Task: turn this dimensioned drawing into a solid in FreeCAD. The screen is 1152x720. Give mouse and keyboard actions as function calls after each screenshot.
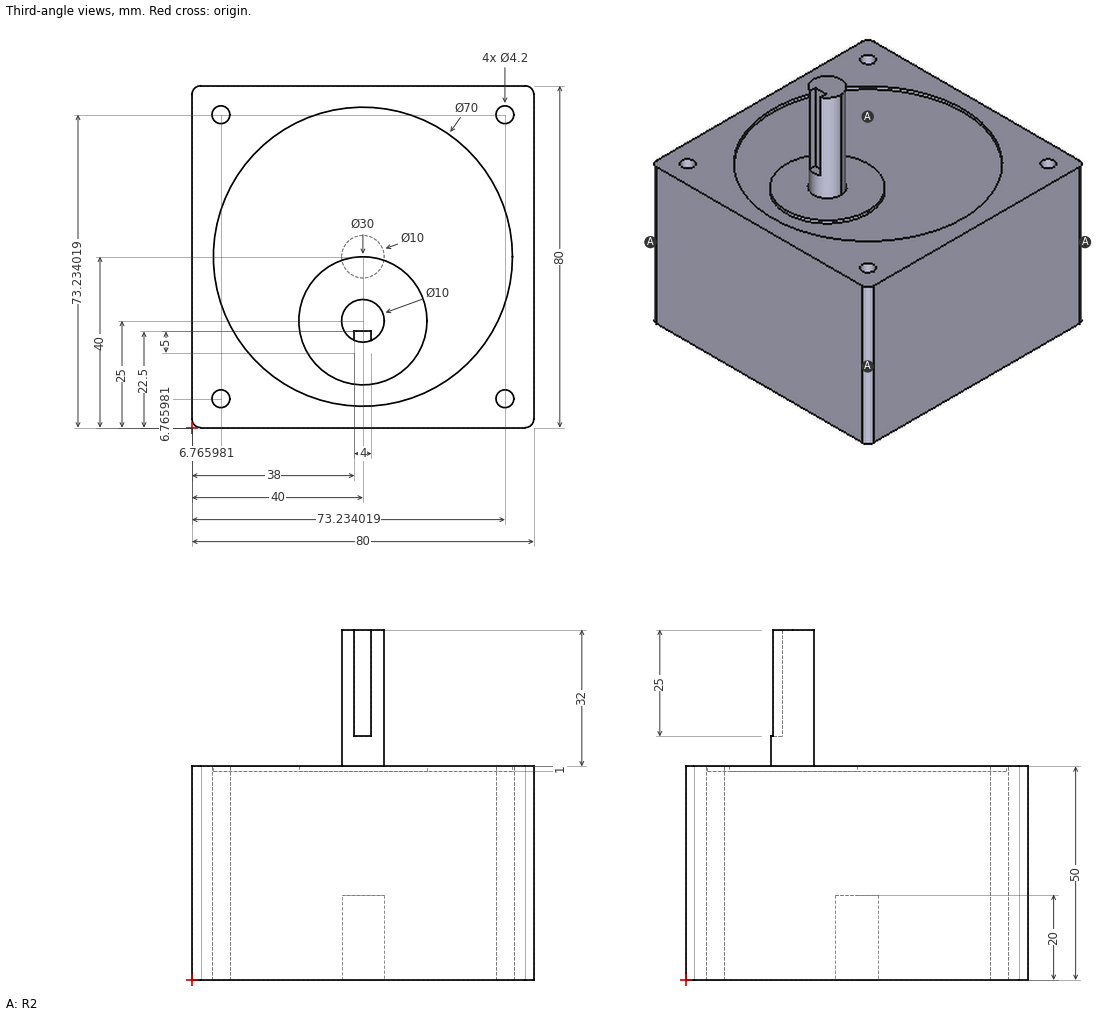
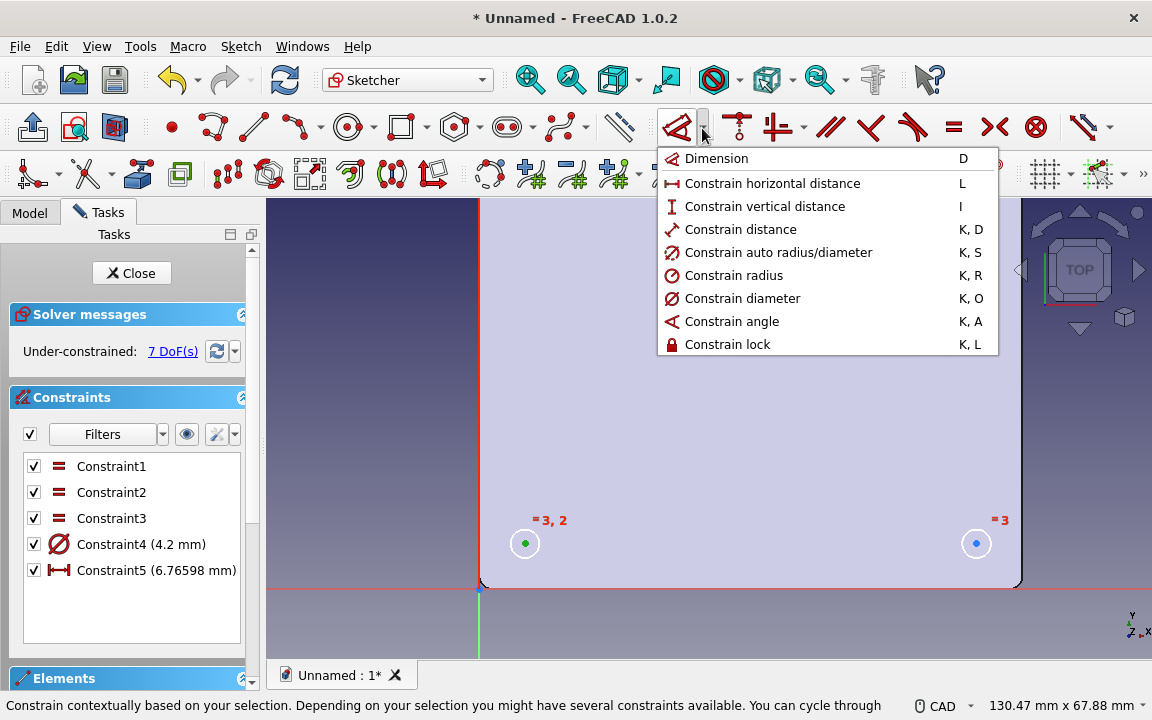
click(828, 184)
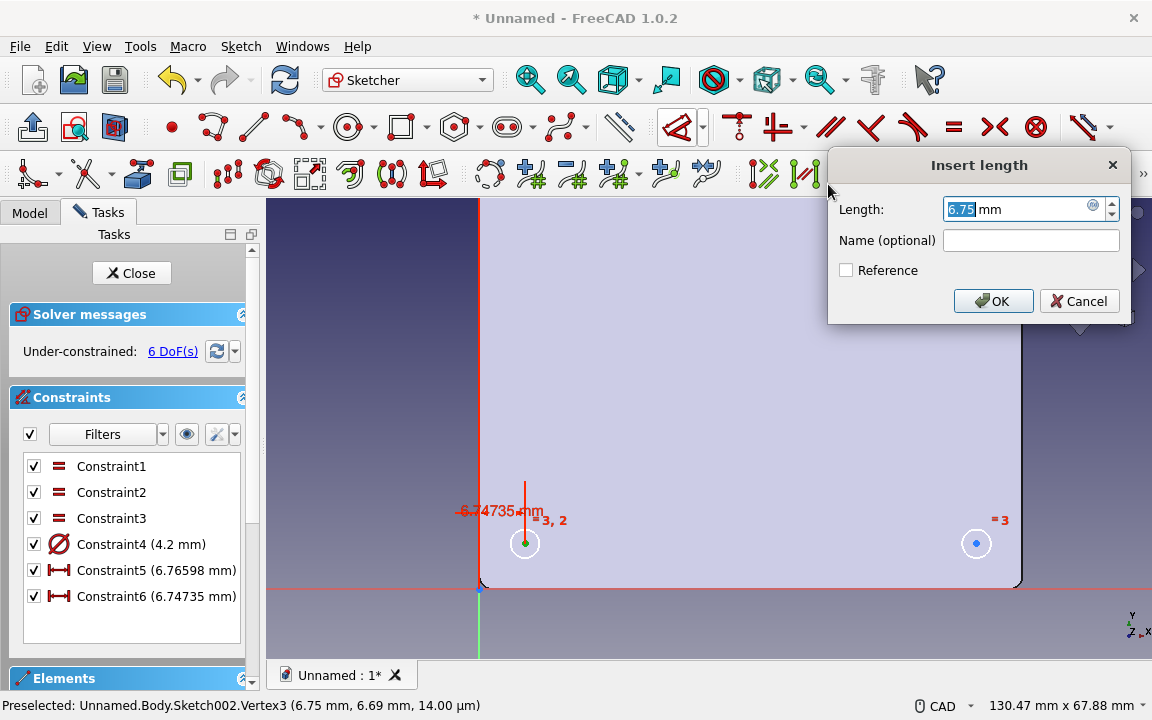
text(6.765981)
key(Return)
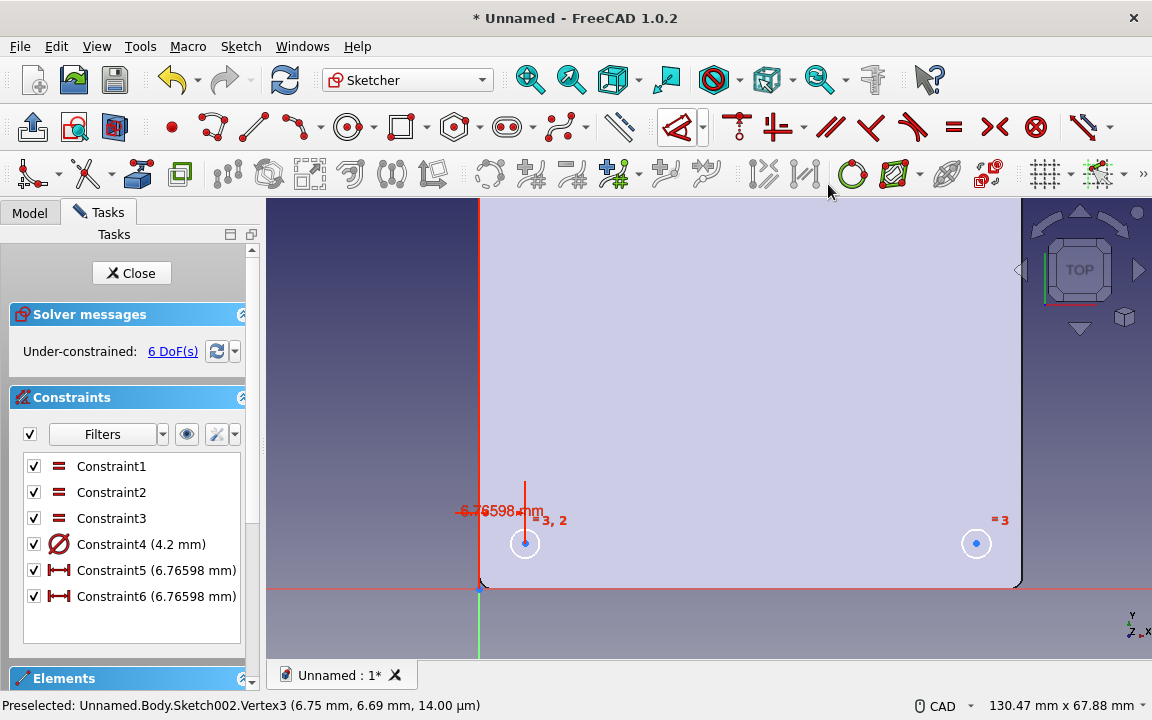
click(525, 544)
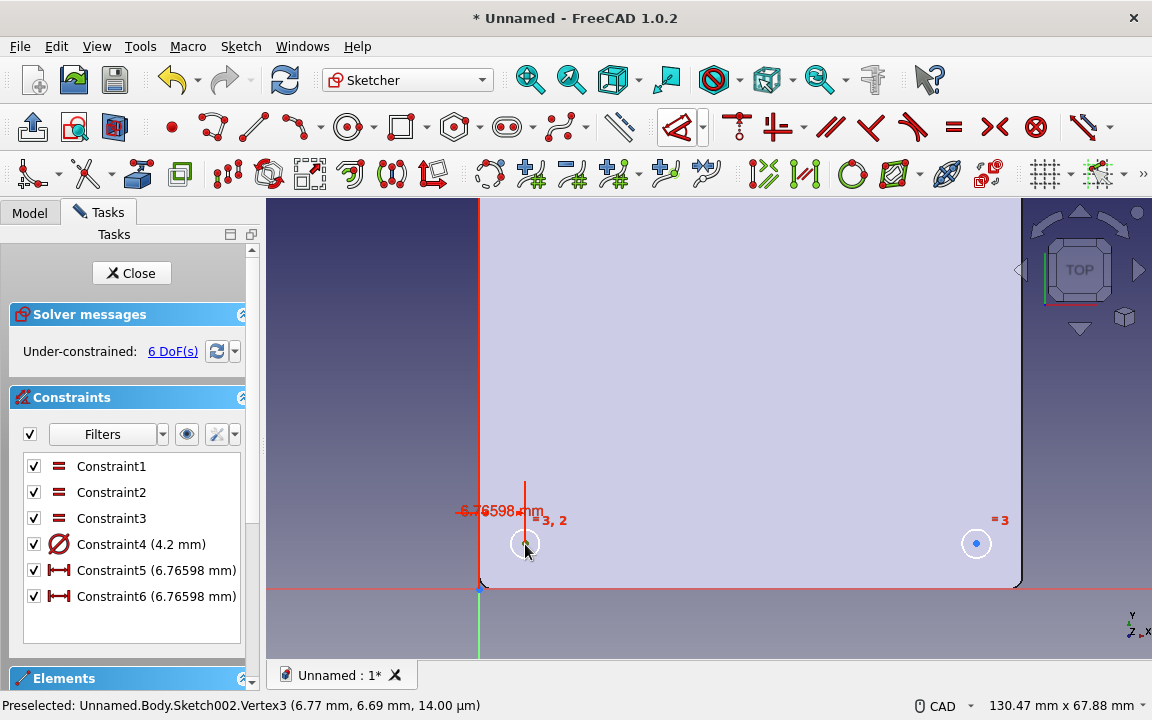
key(i)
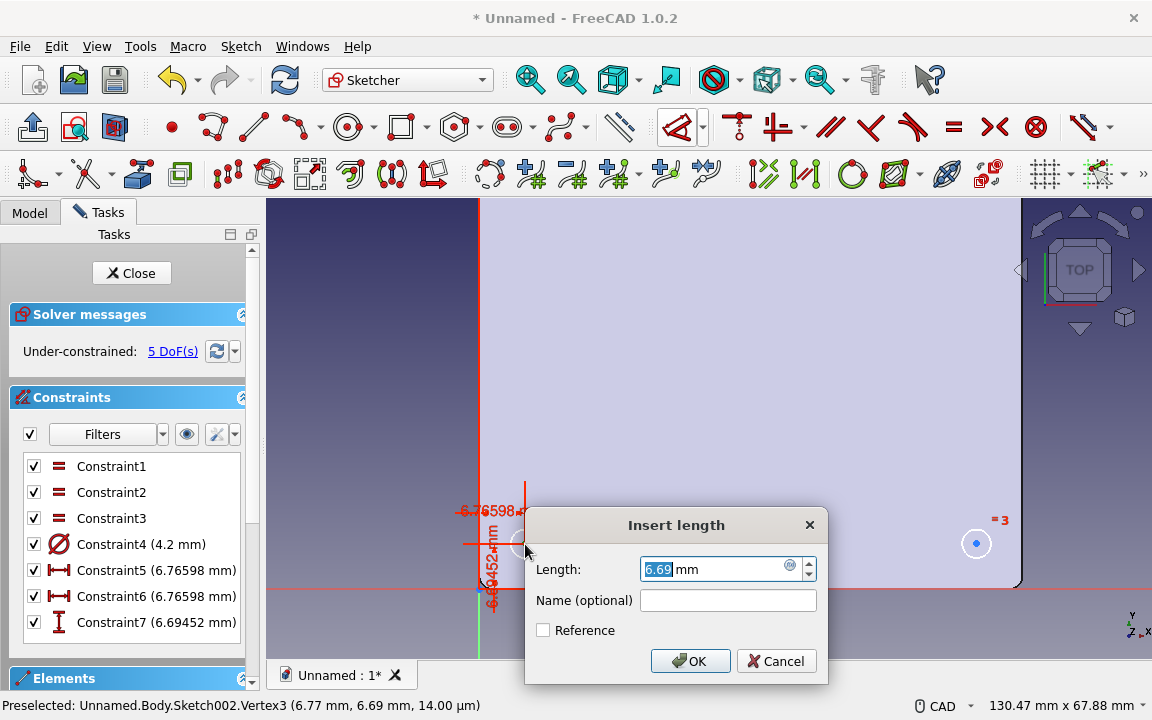
text(6.765981)
key(Return)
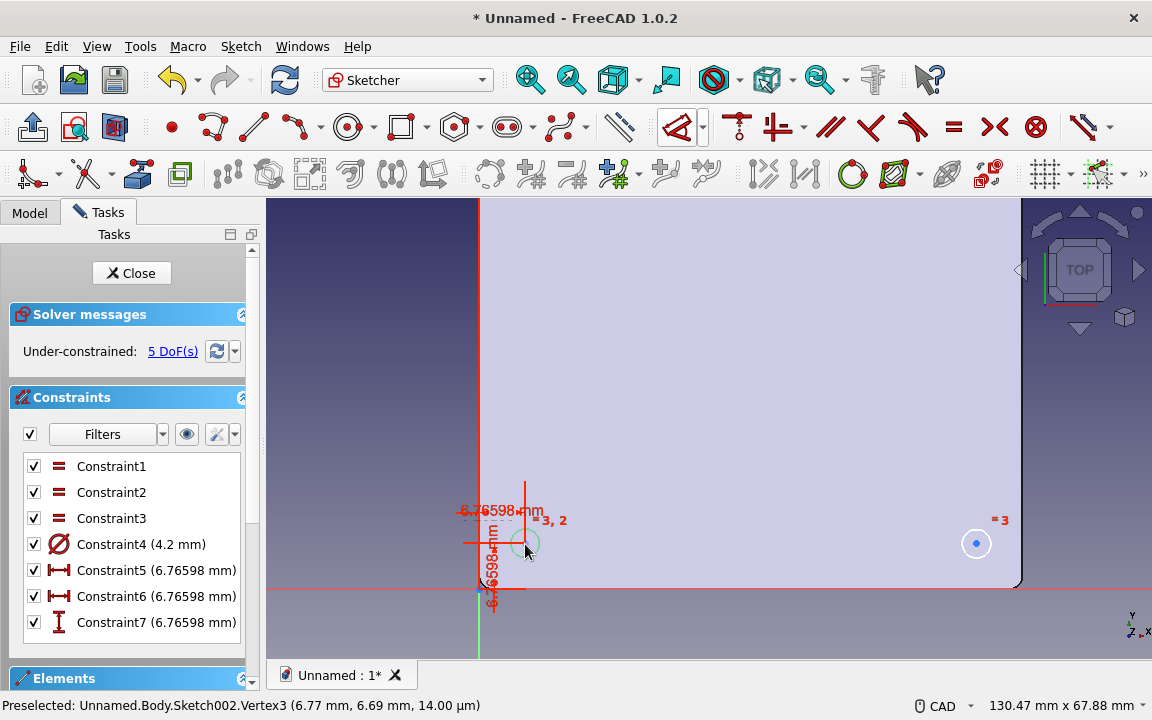
click(977, 544)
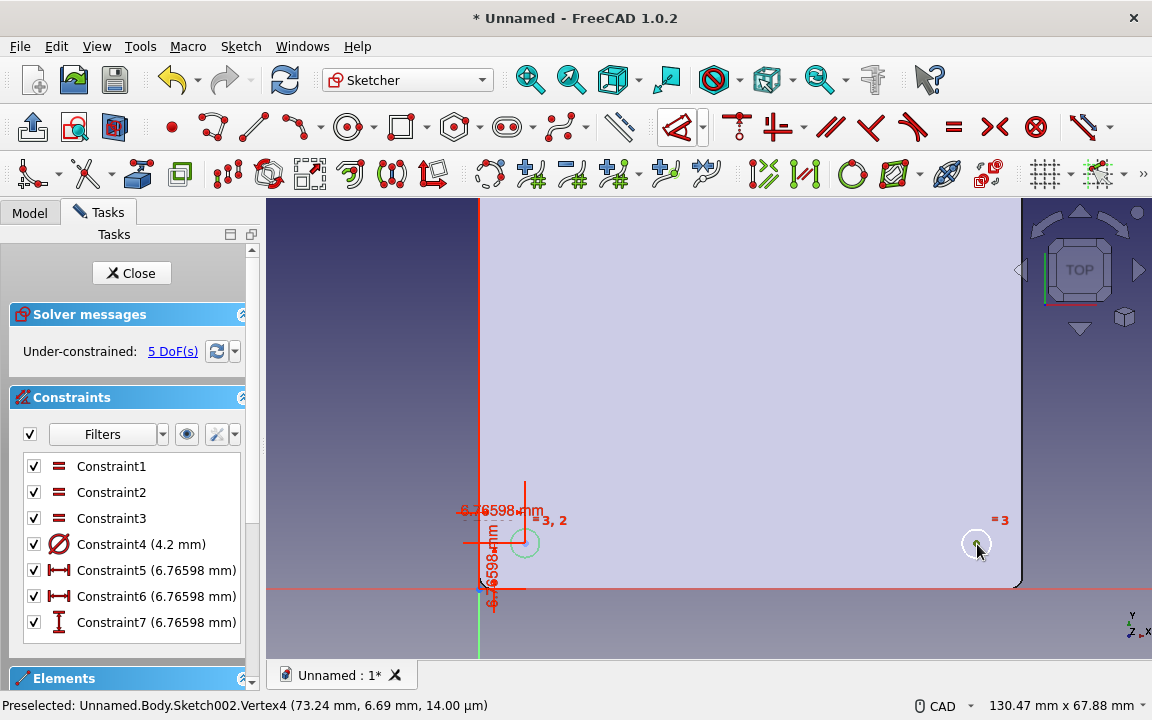
key(i)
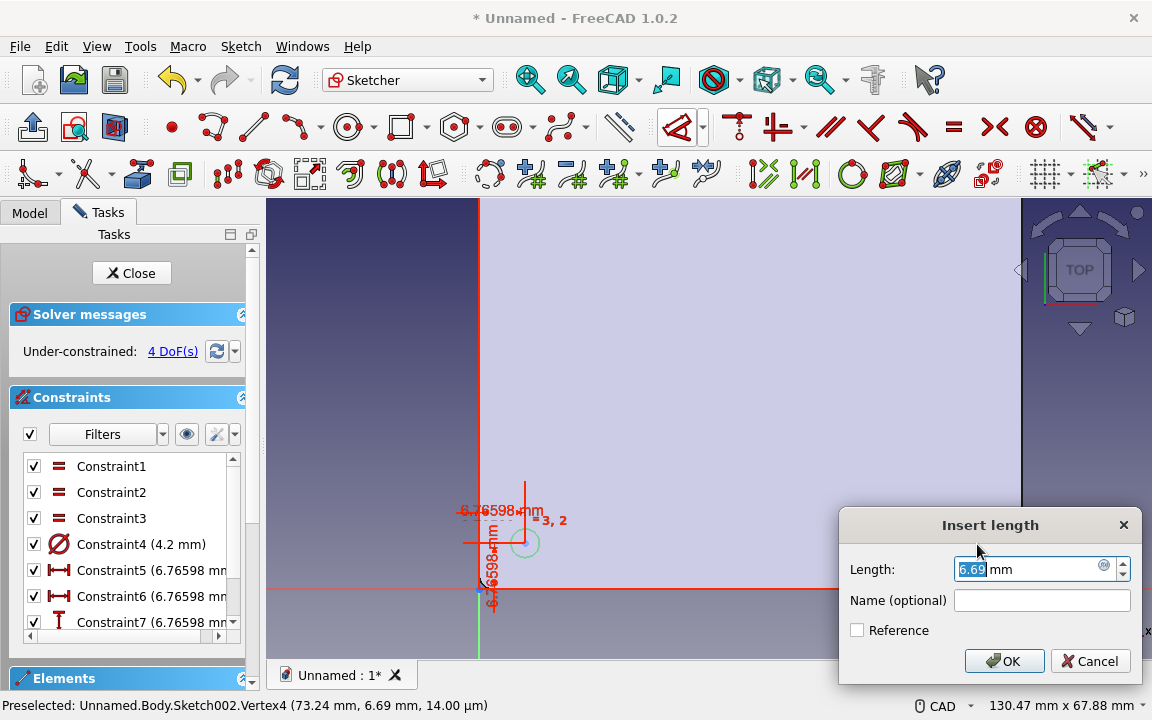
text(6.765981)
key(Return)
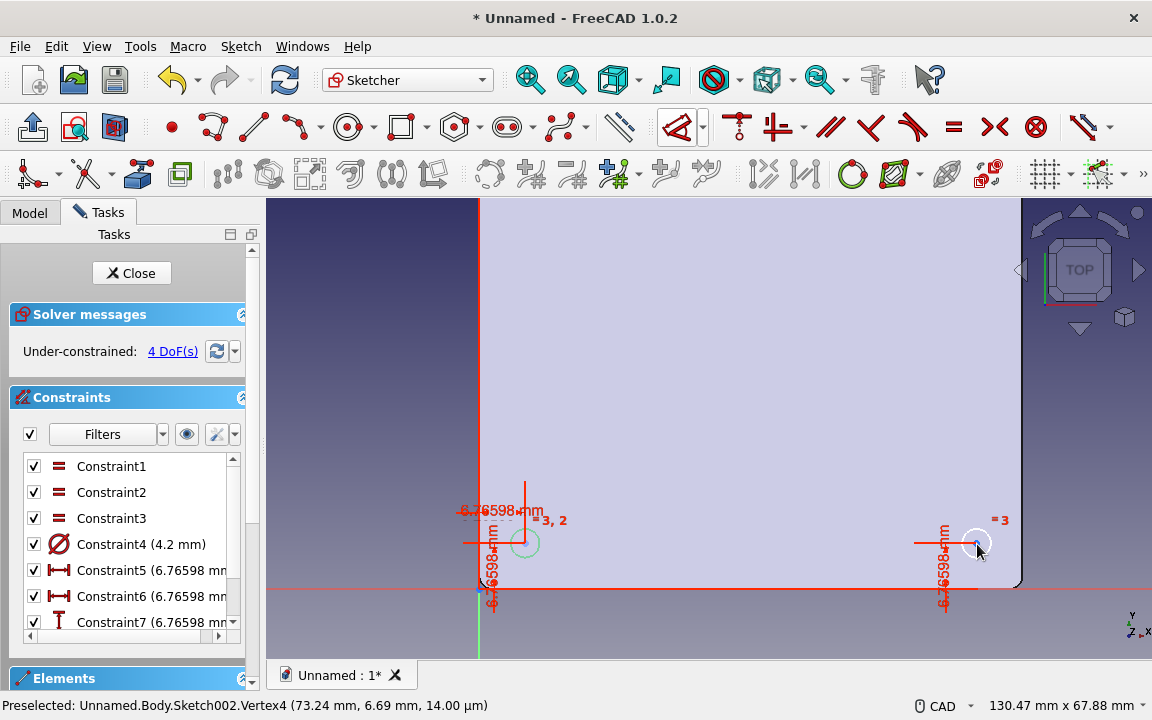
scroll(526, 544, down, 3)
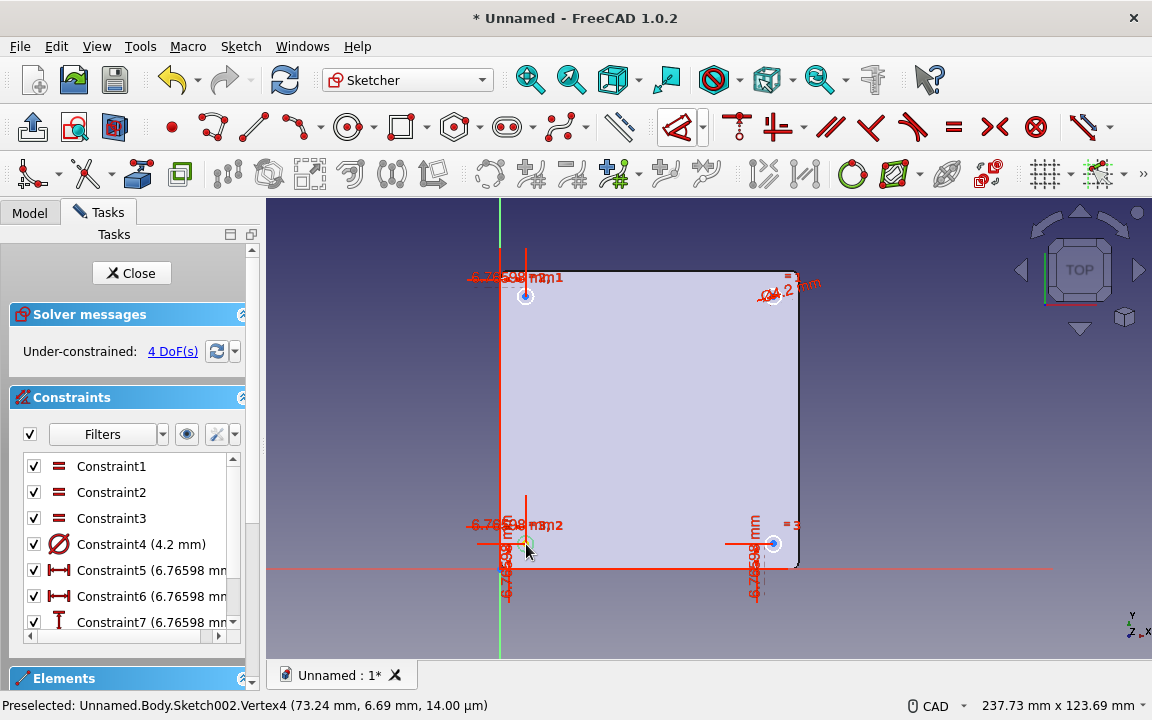
click(773, 296)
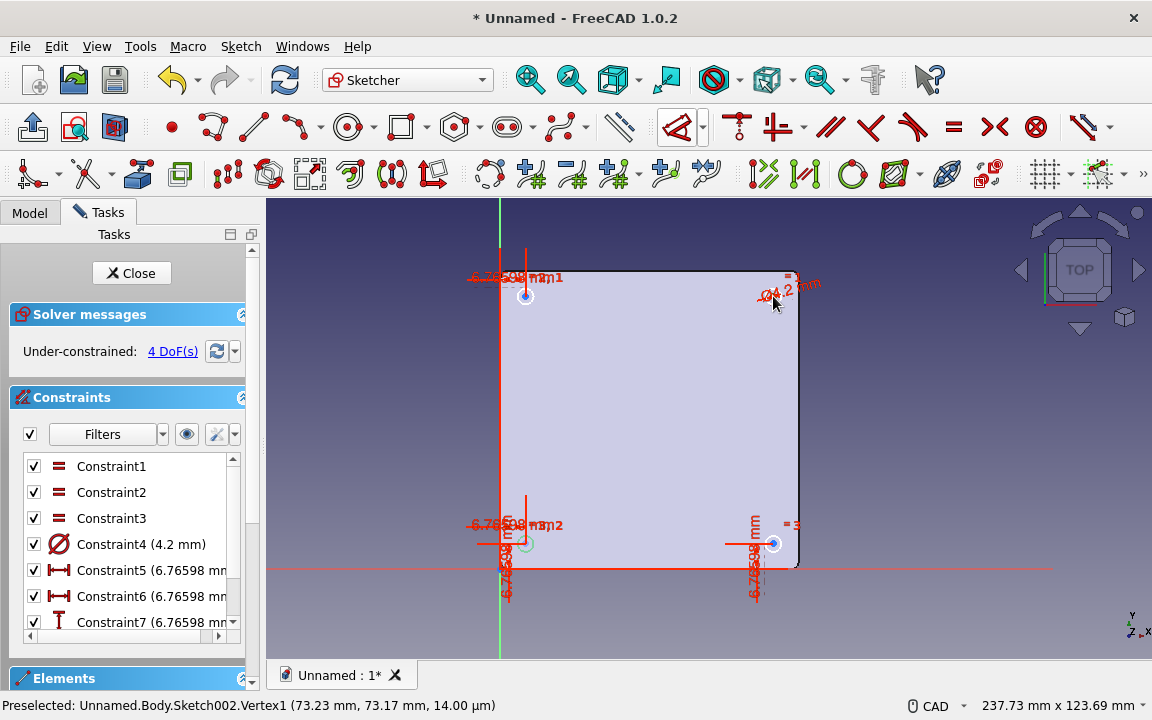
click(702, 128)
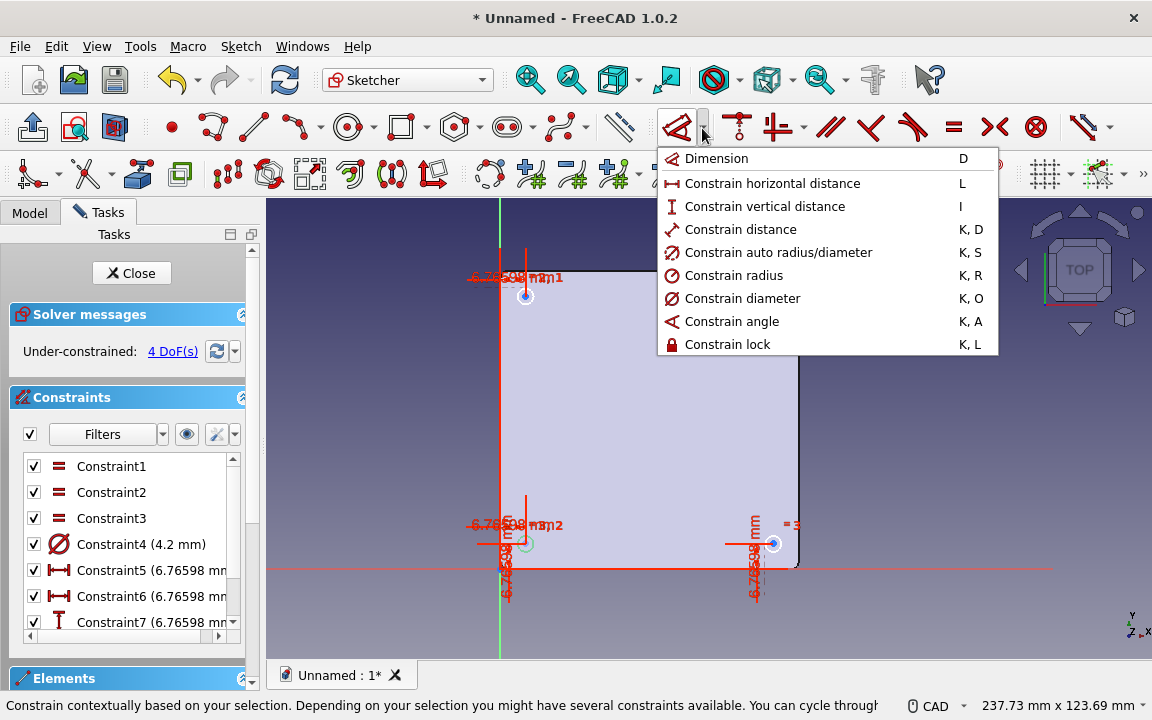
click(828, 184)